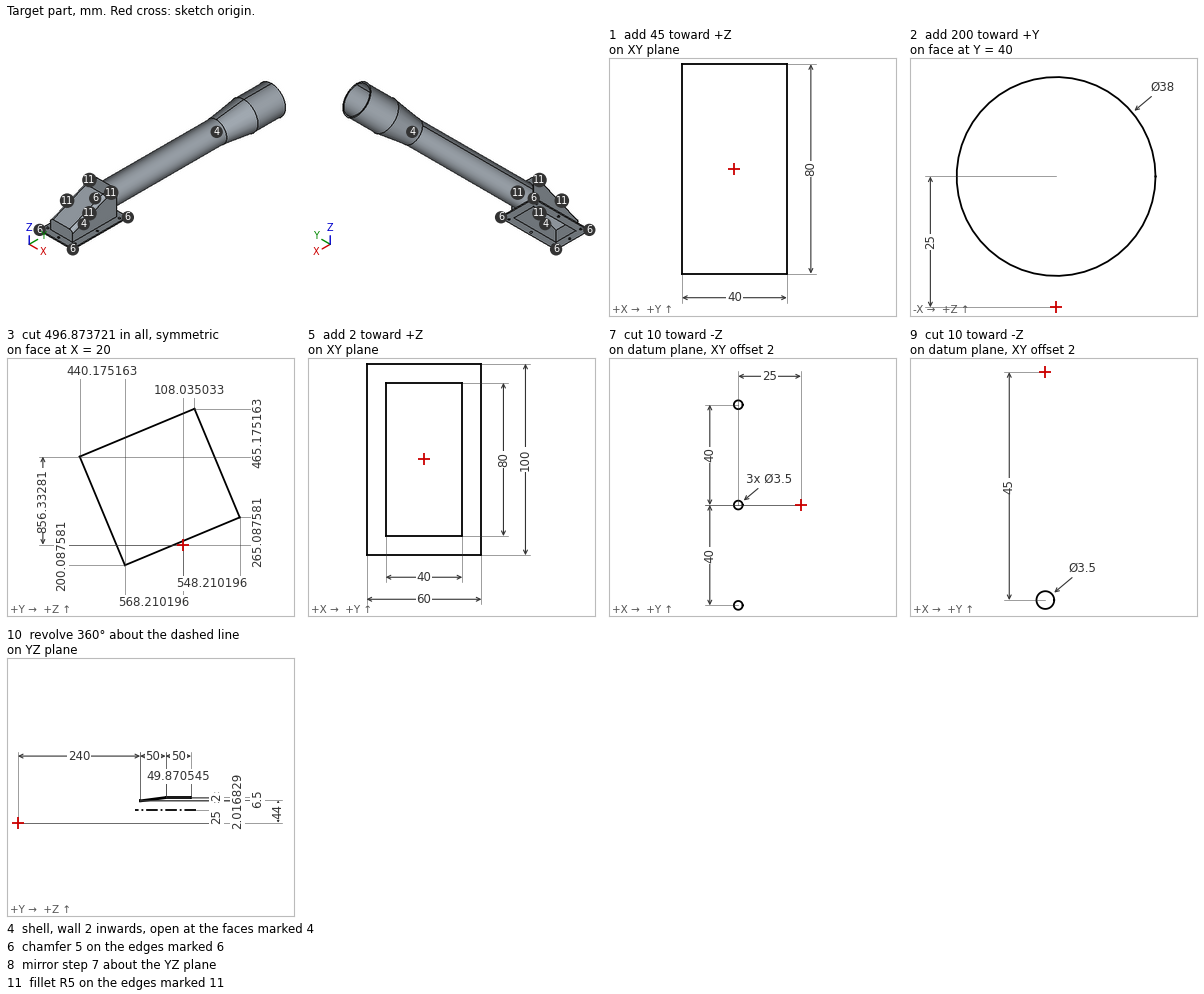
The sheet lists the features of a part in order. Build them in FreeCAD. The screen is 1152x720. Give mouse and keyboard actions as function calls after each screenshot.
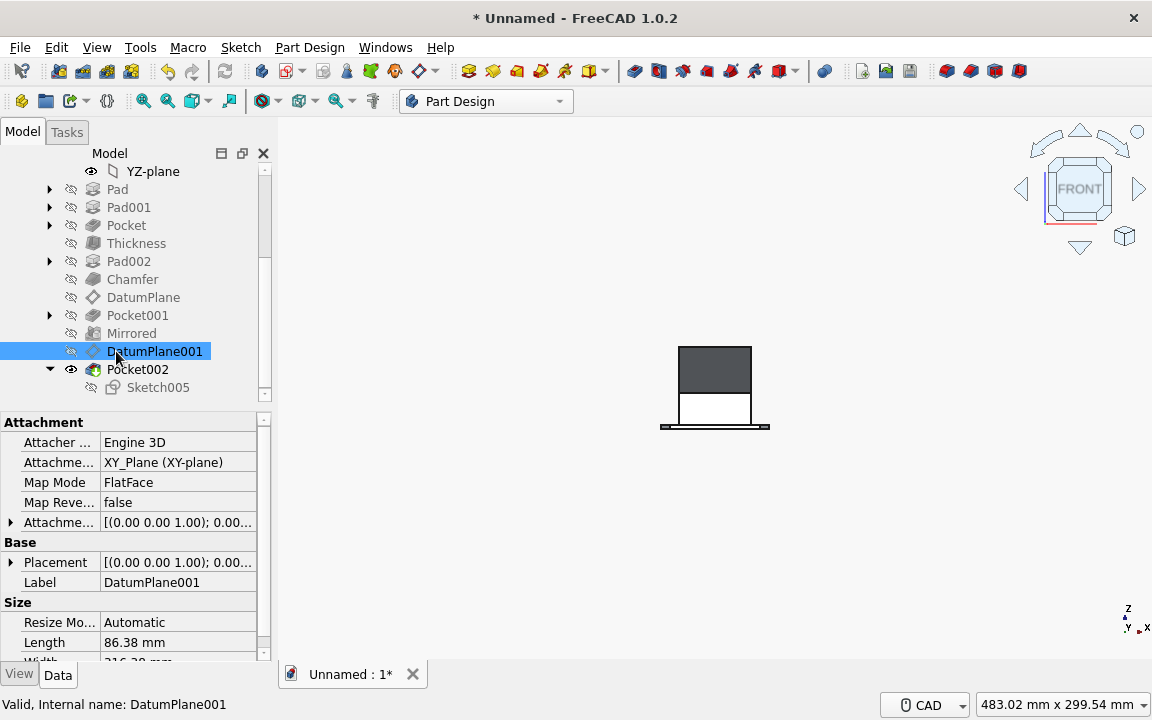
click(318, 619)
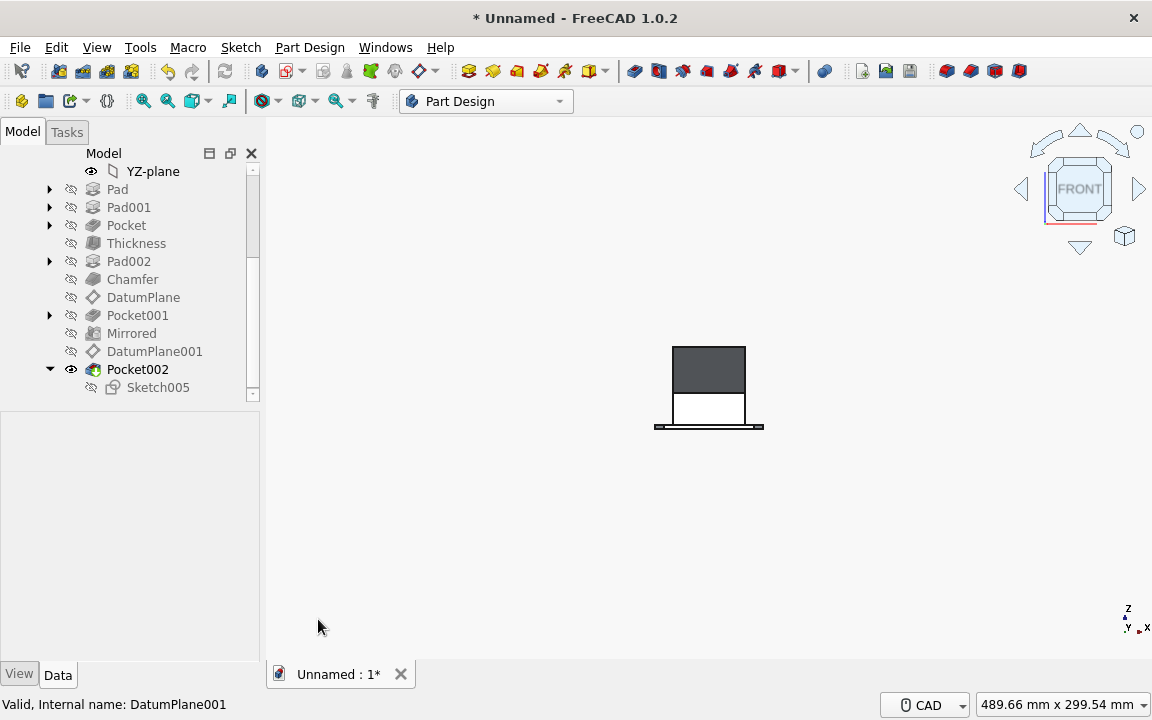
click(286, 72)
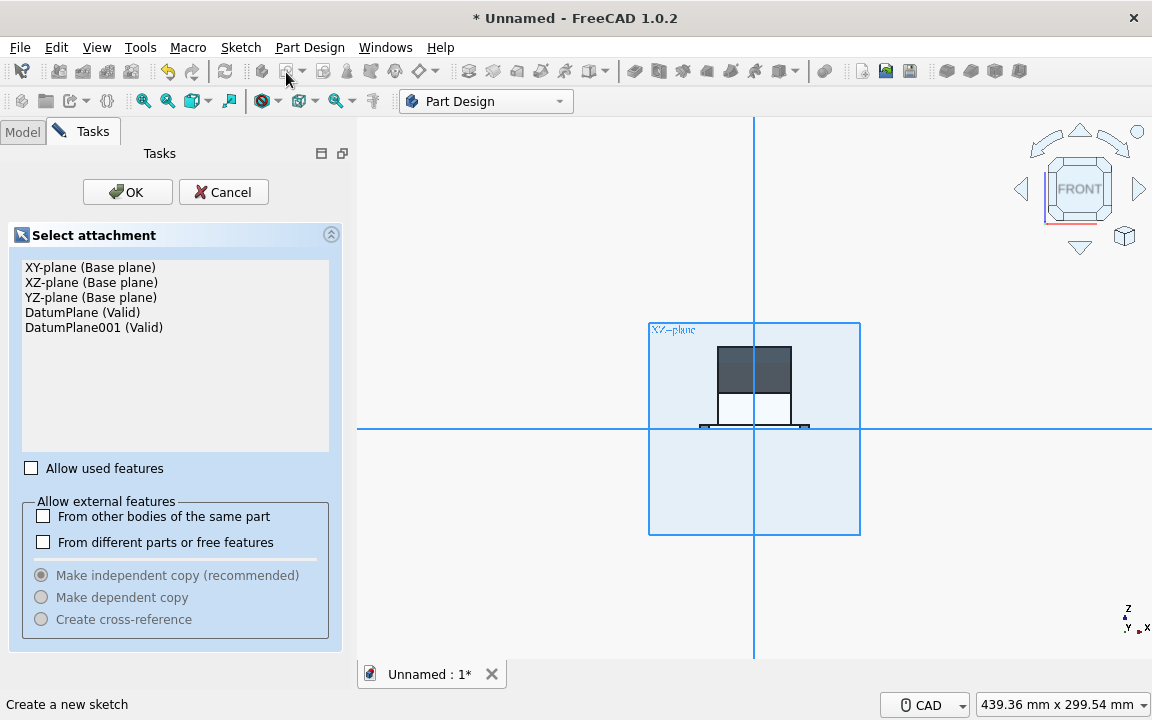
click(82, 298)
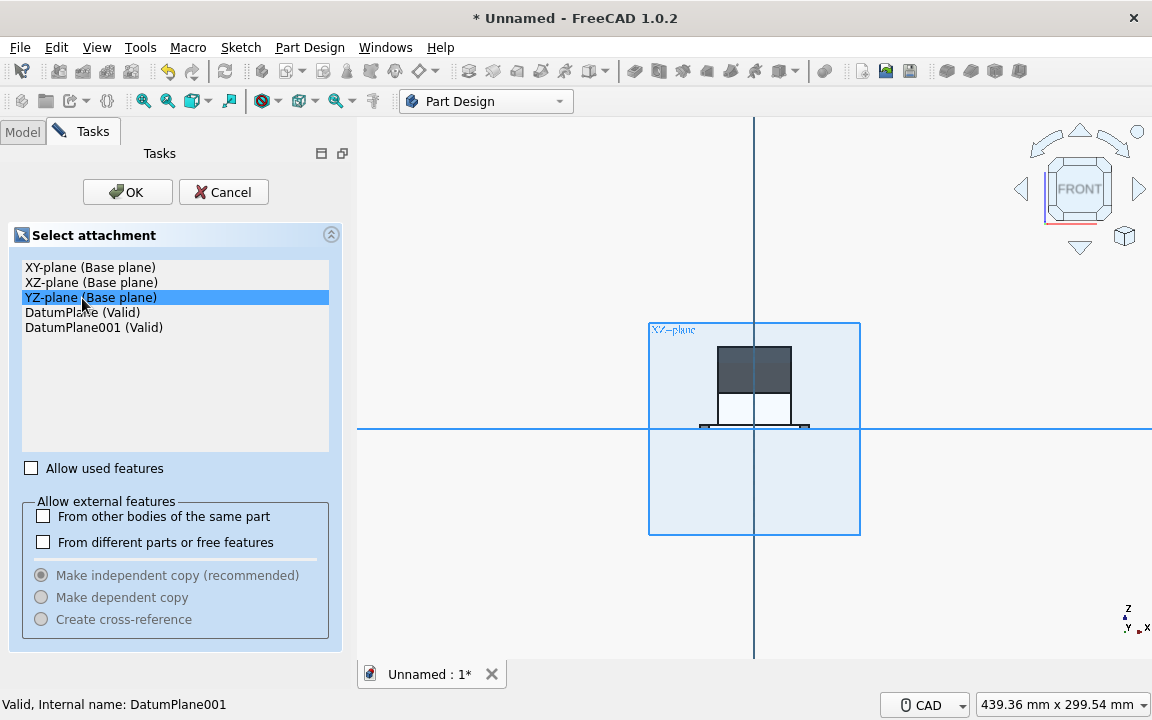
click(128, 192)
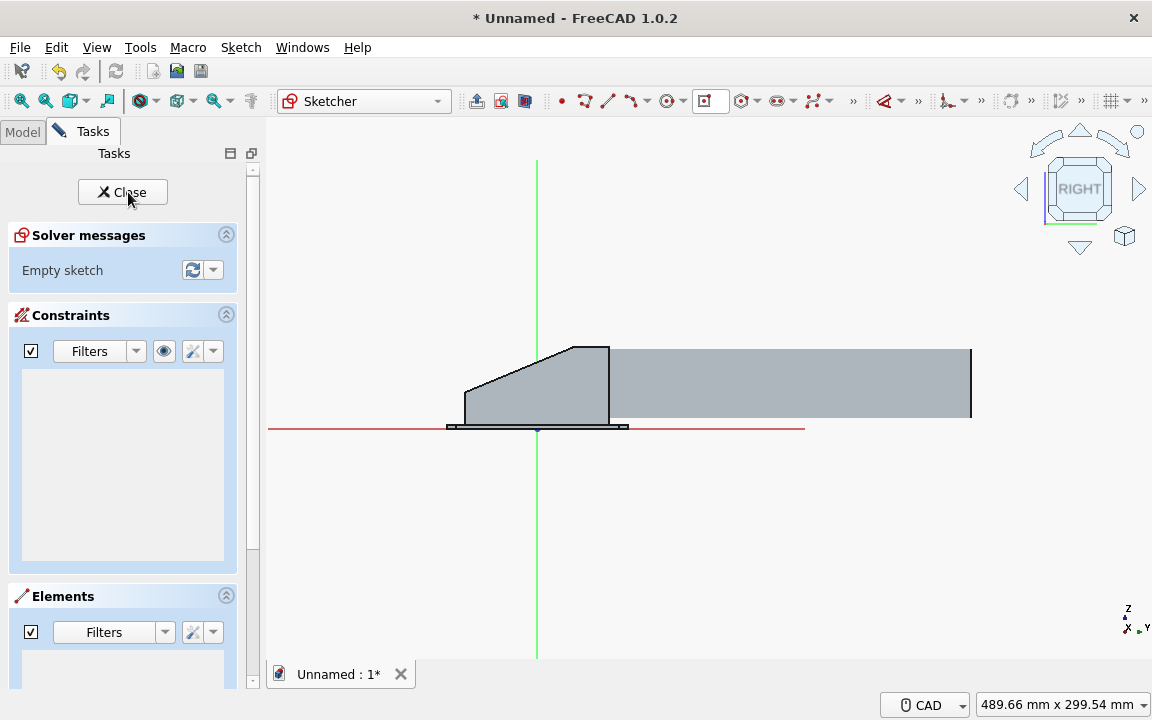
key(q)
key(s)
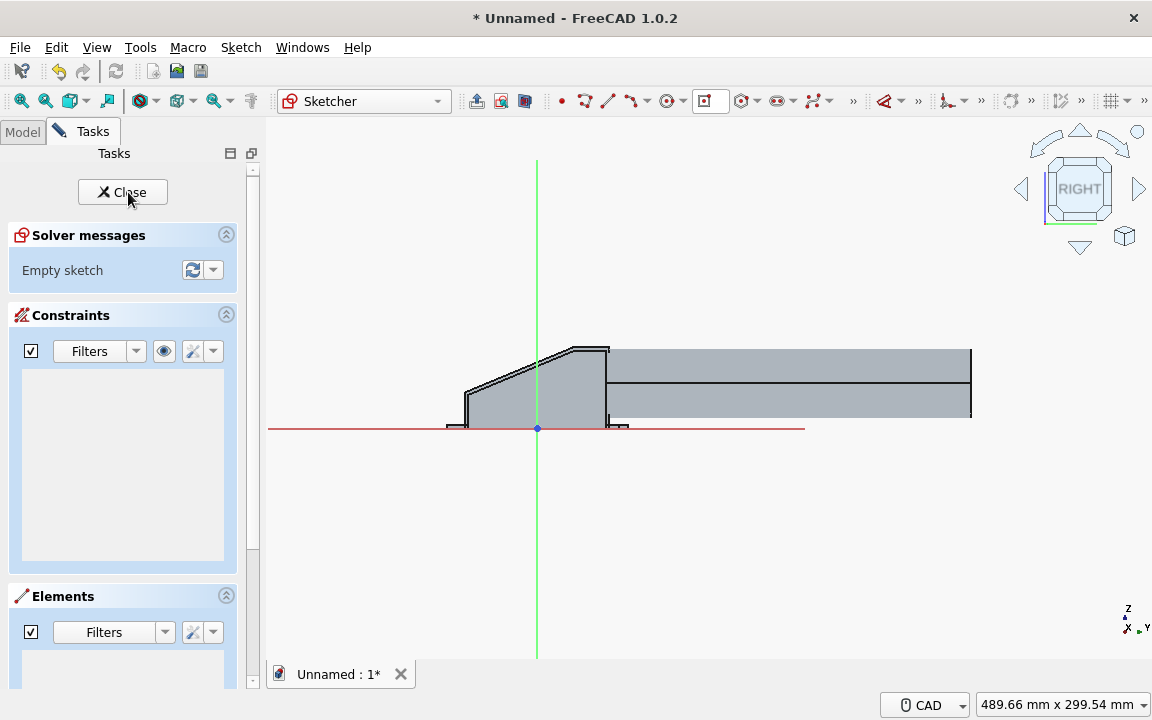
scroll(640, 388, down, 5)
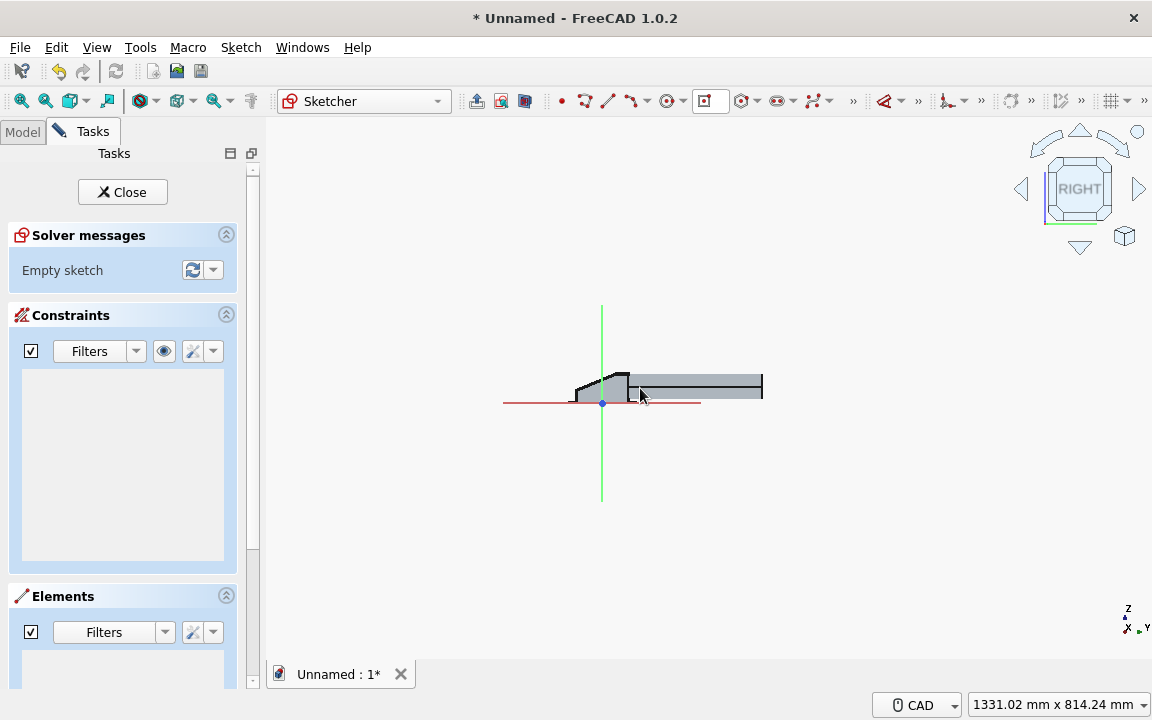
scroll(826, 376, up, 9)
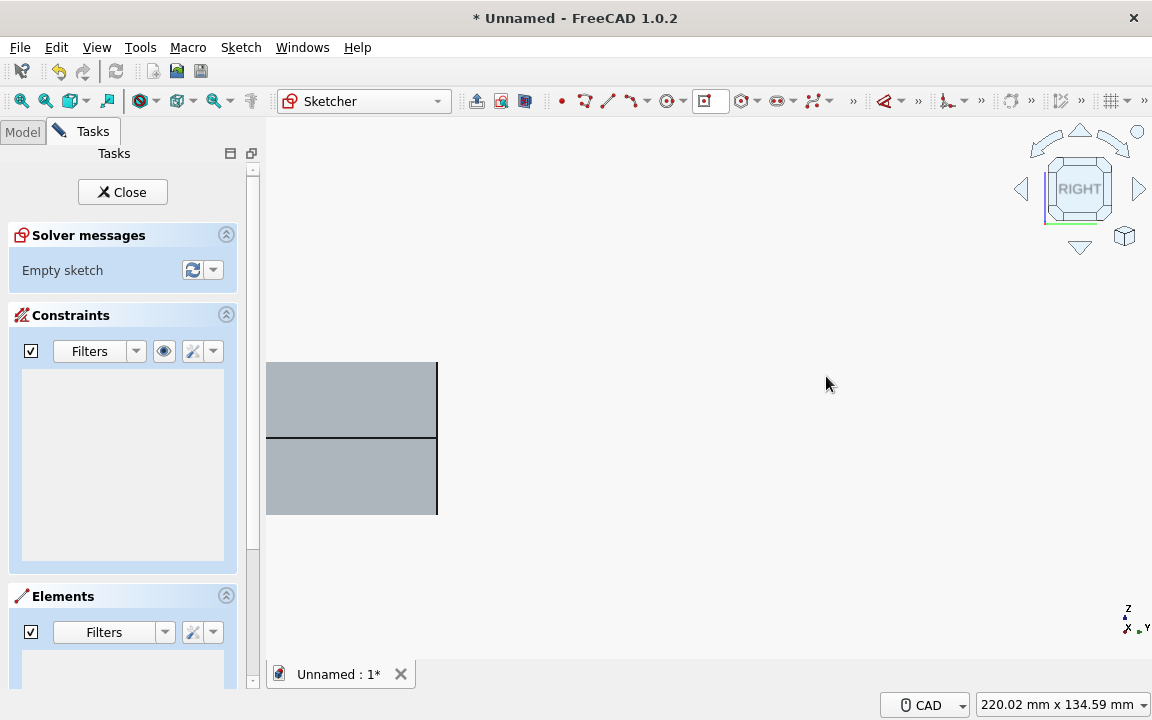
click(586, 102)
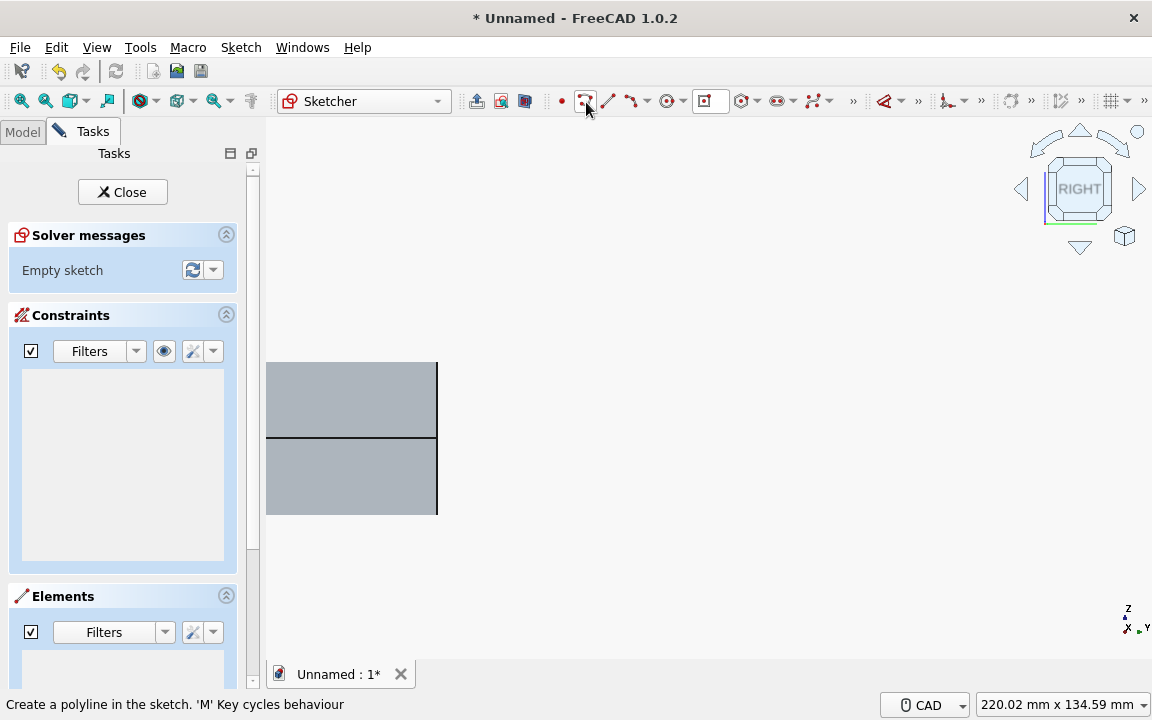
click(437, 370)
click(639, 343)
click(839, 343)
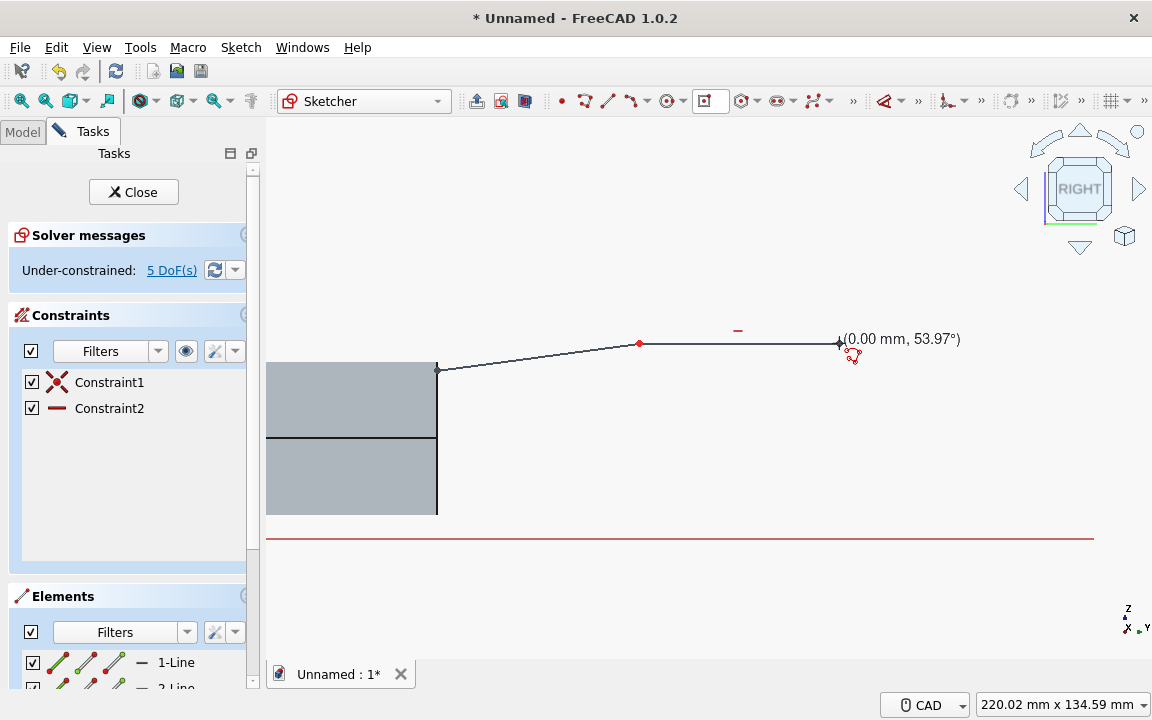
scroll(839, 335, up, 4)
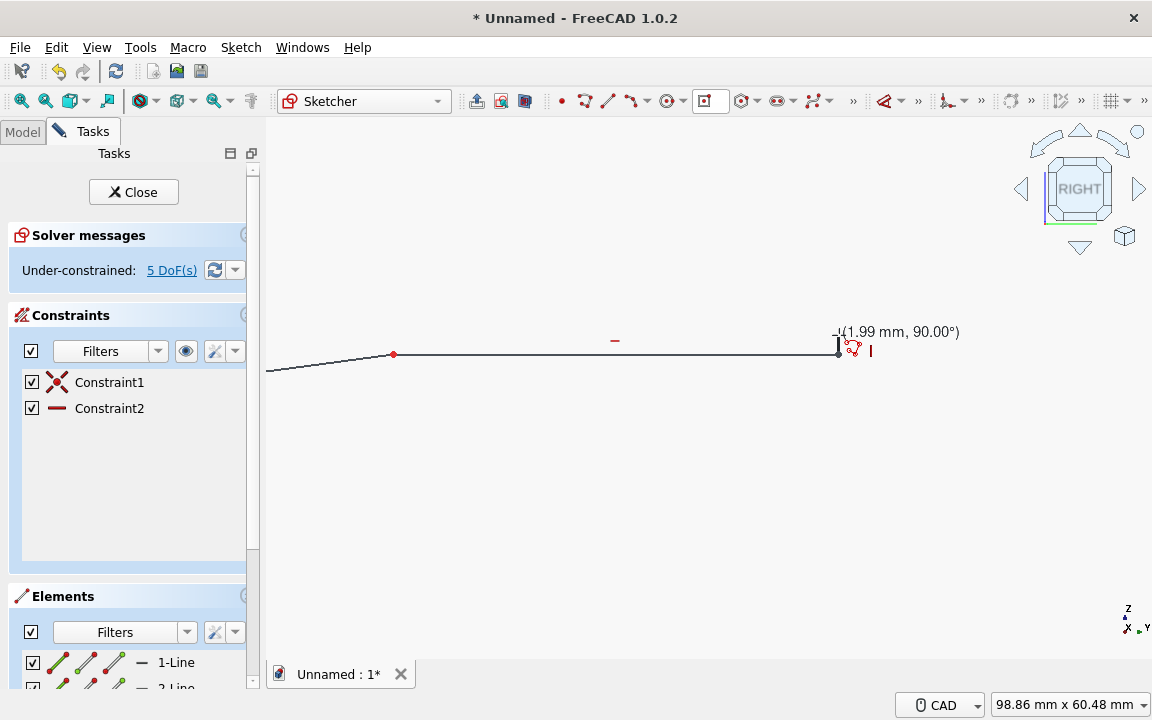
click(838, 335)
click(391, 335)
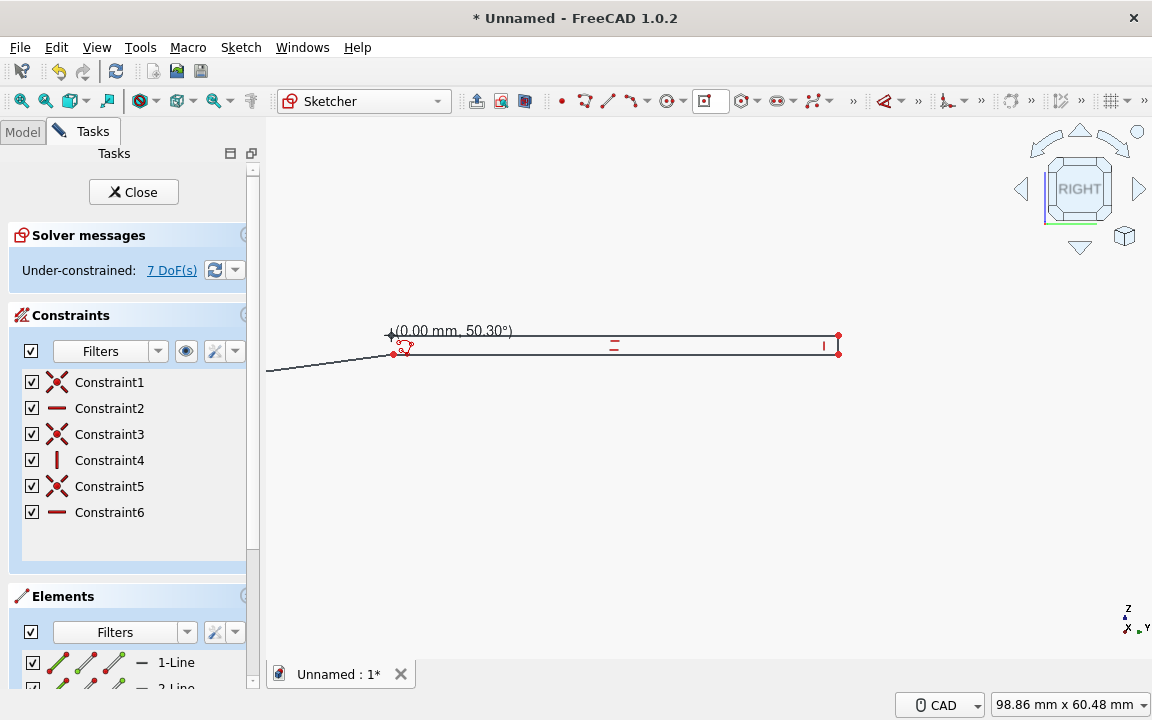
scroll(844, 338, down, 4)